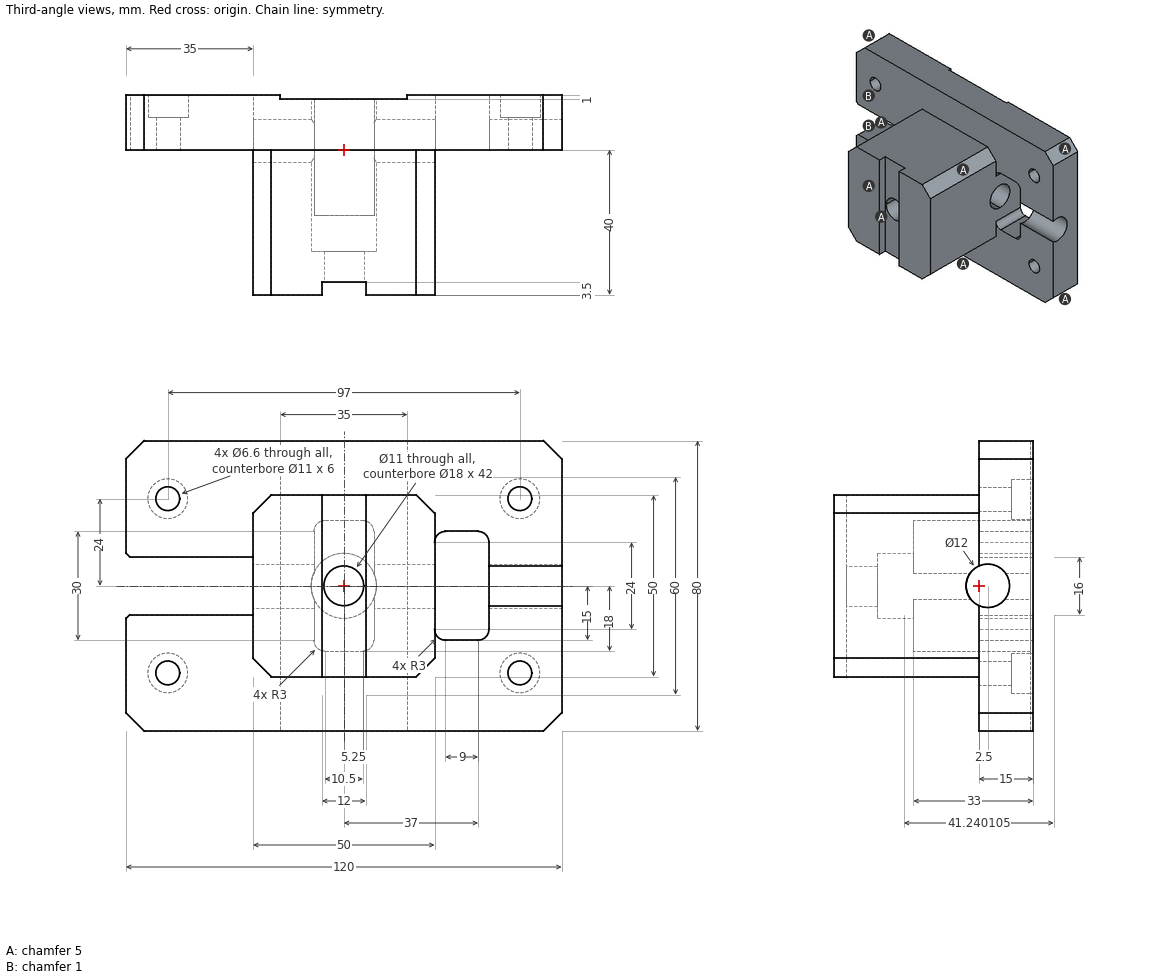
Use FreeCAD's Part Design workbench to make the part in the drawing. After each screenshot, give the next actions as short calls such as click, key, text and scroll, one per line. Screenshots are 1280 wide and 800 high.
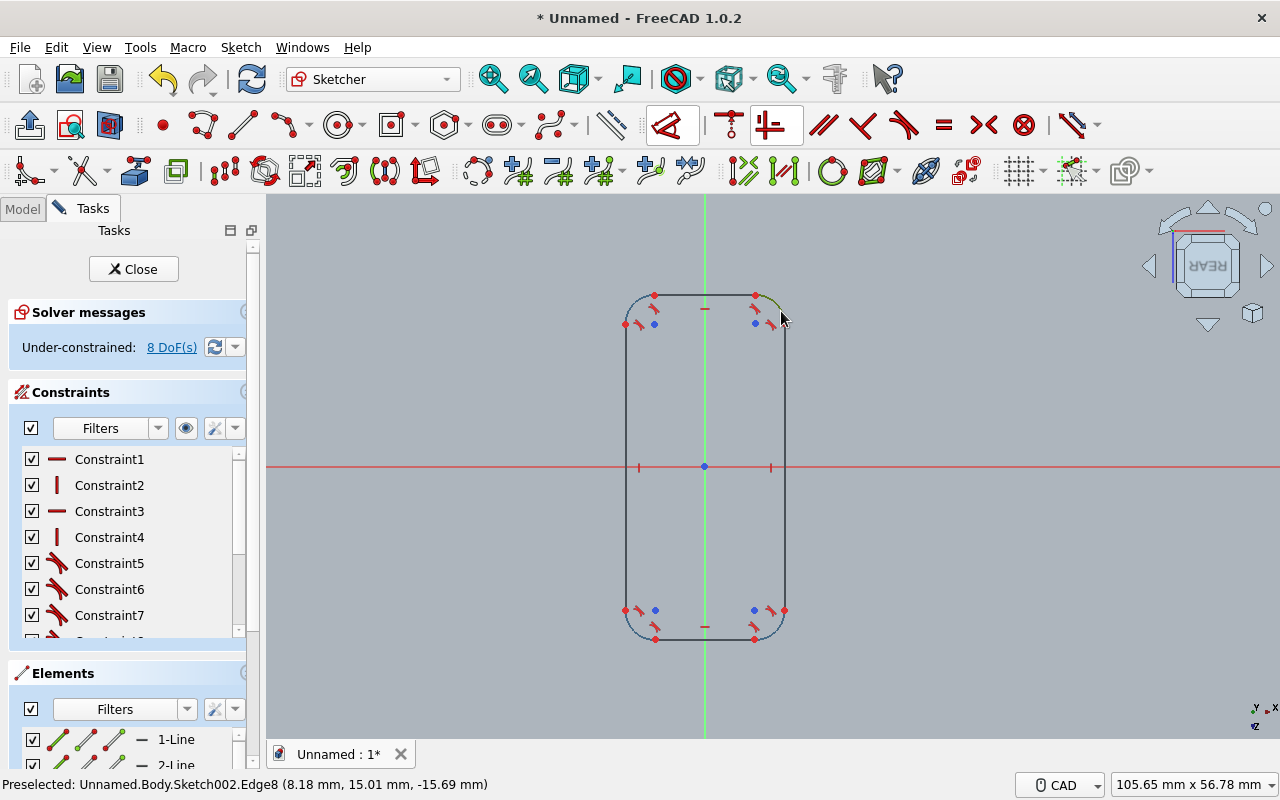
click(944, 126)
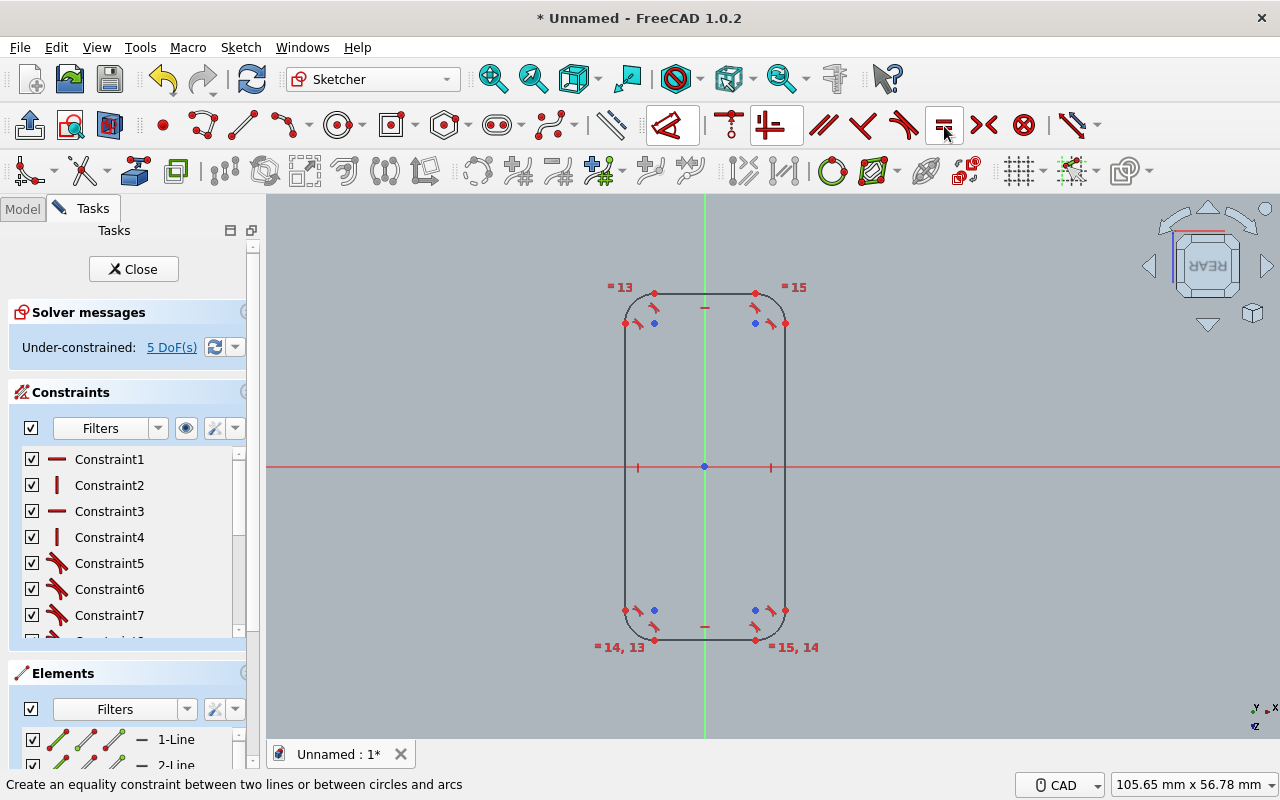
scroll(641, 297, up, 2)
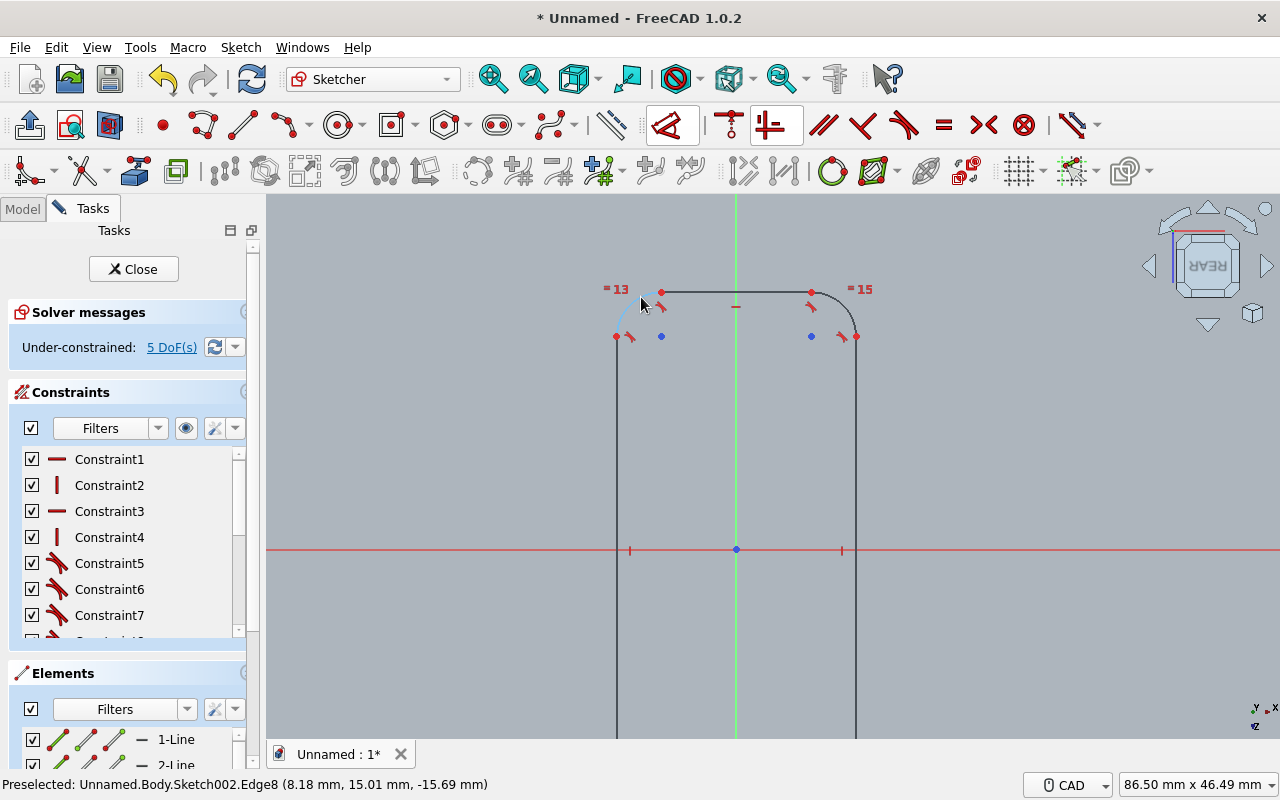
click(641, 297)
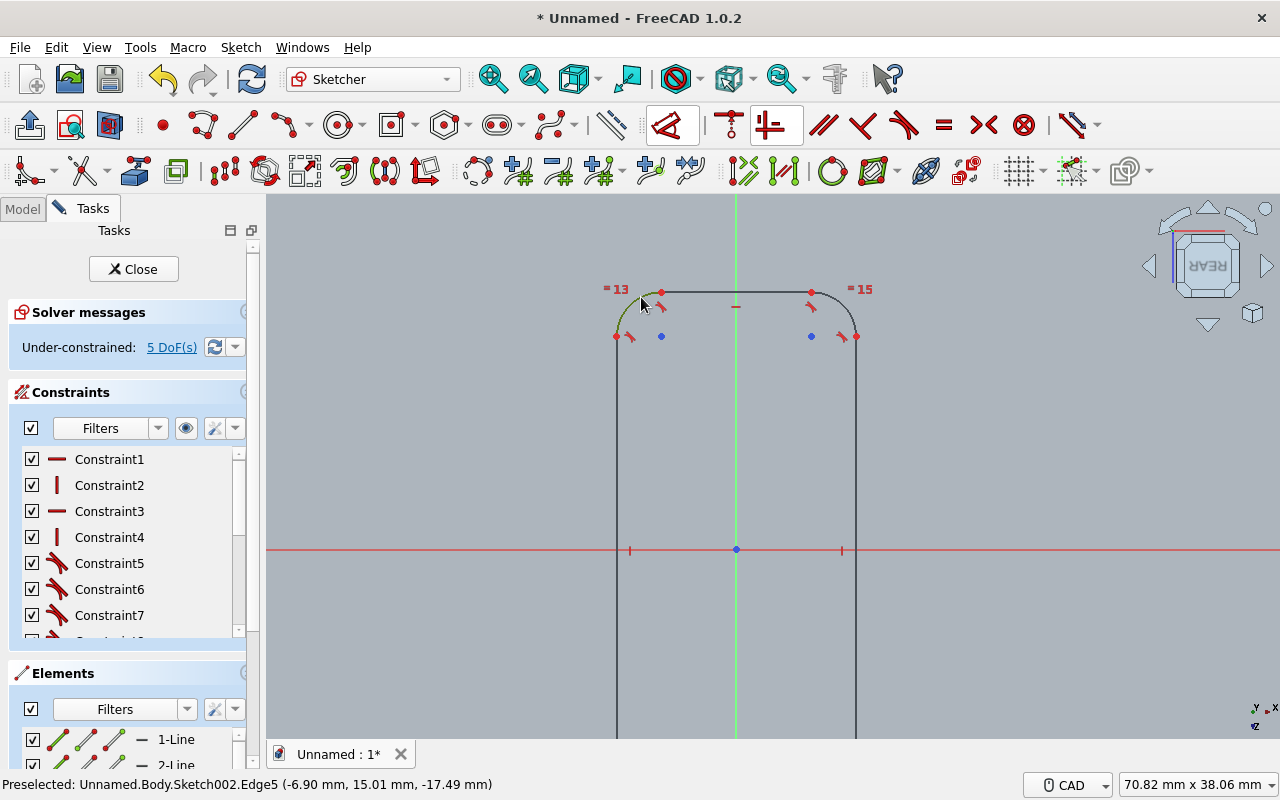
key(k)
key(r)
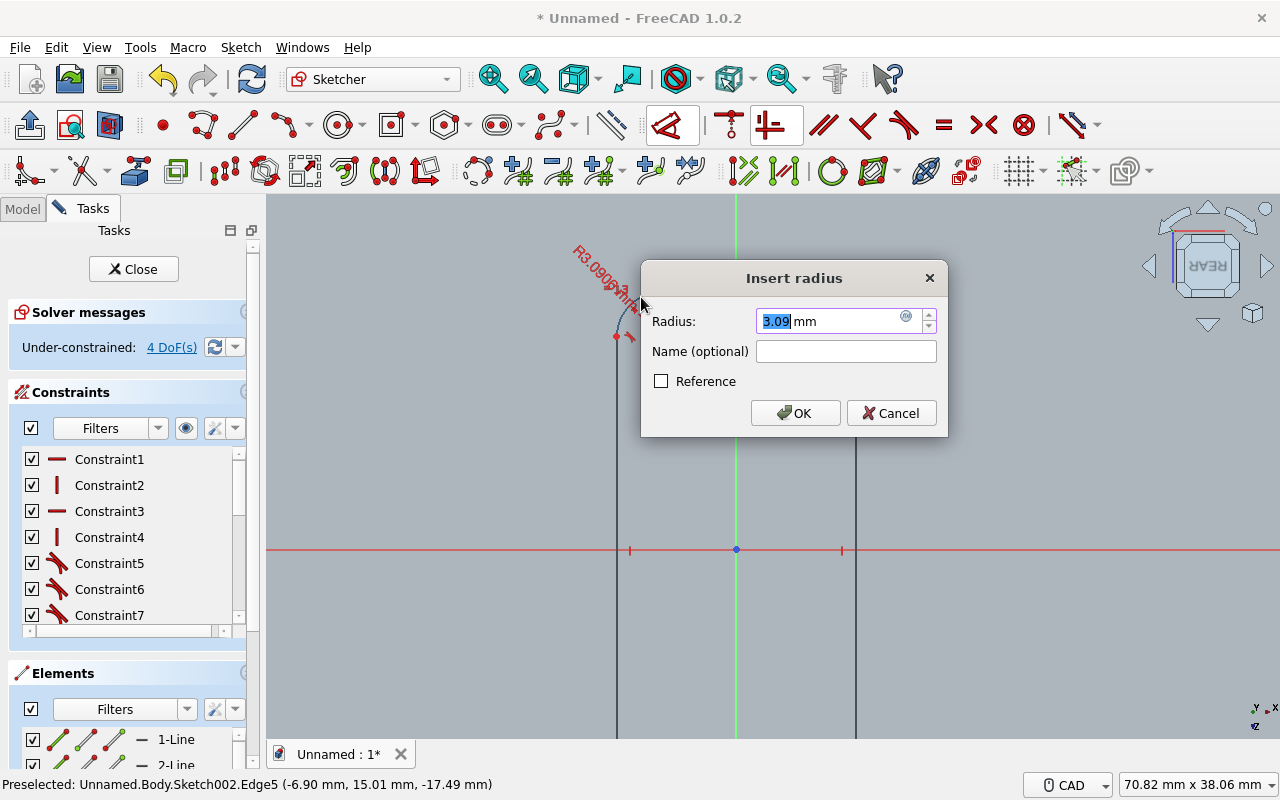
text(3)
key(Return)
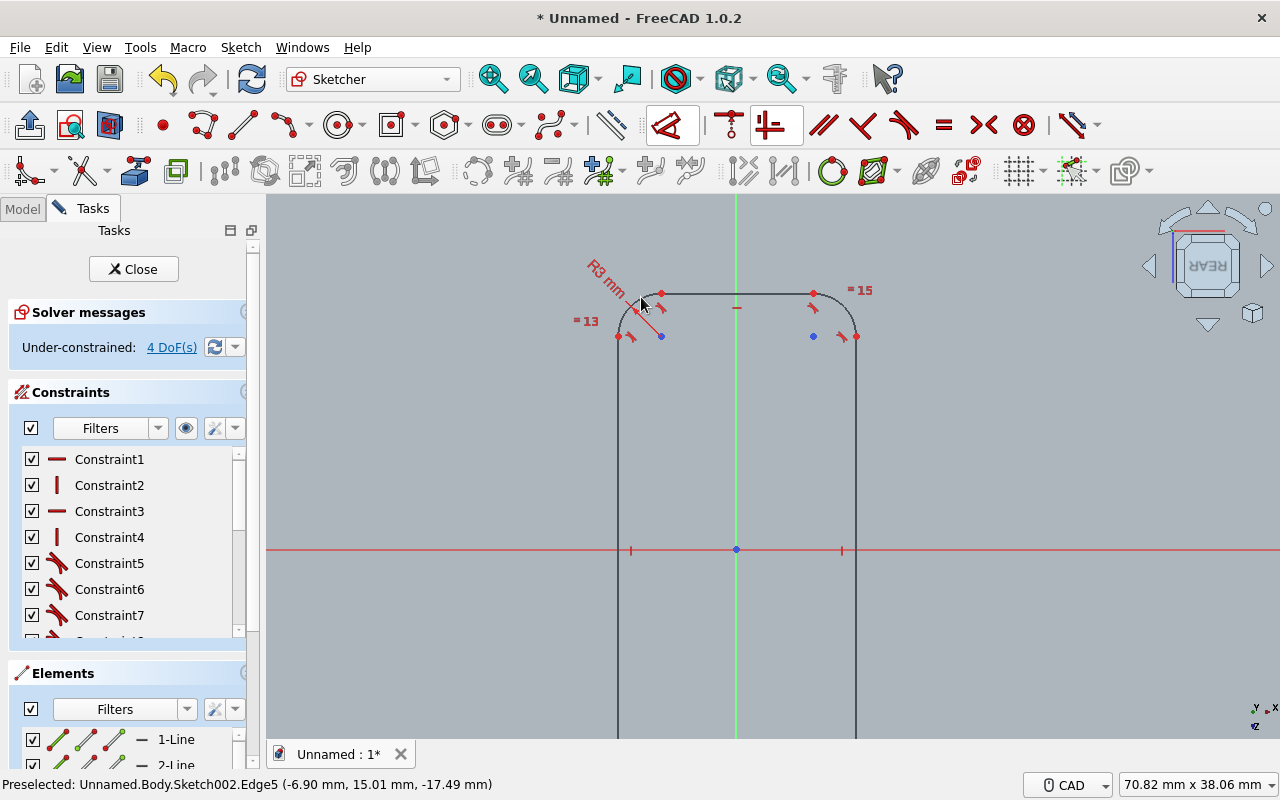
click(618, 465)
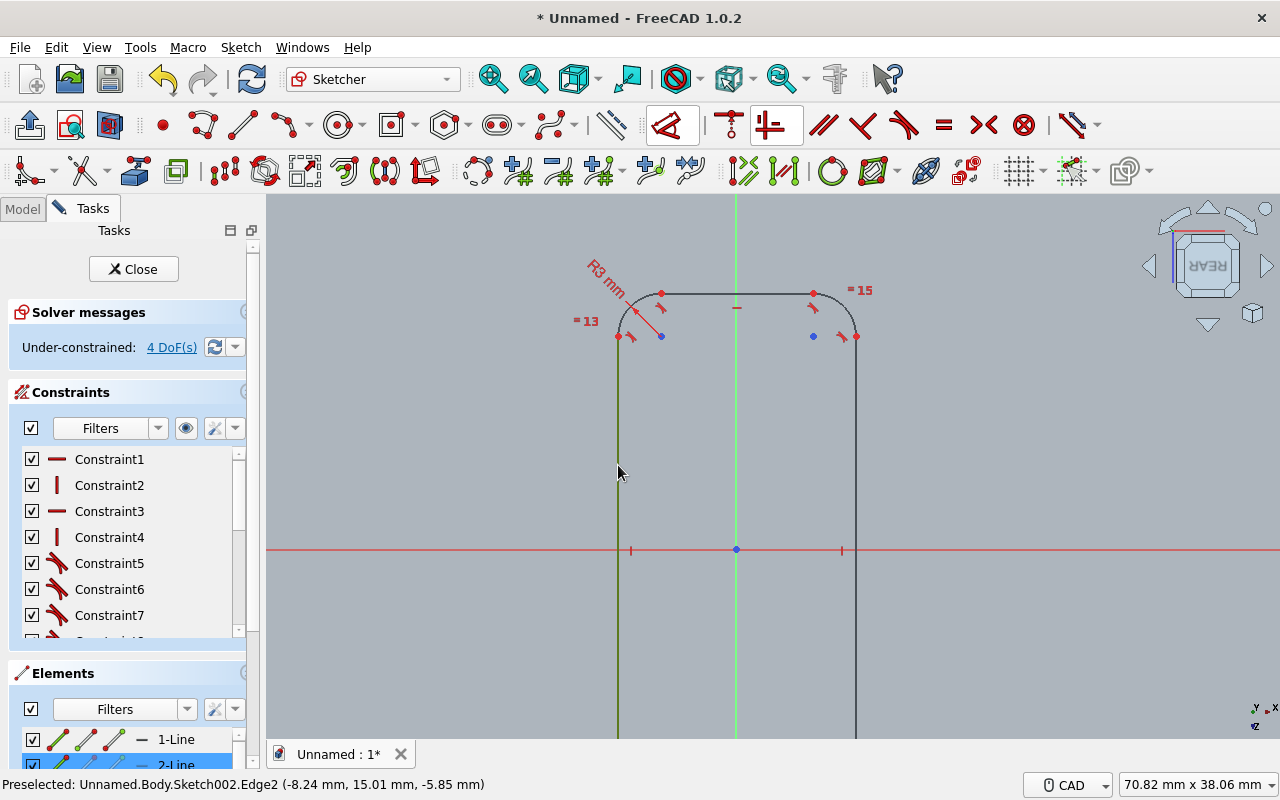
key(i)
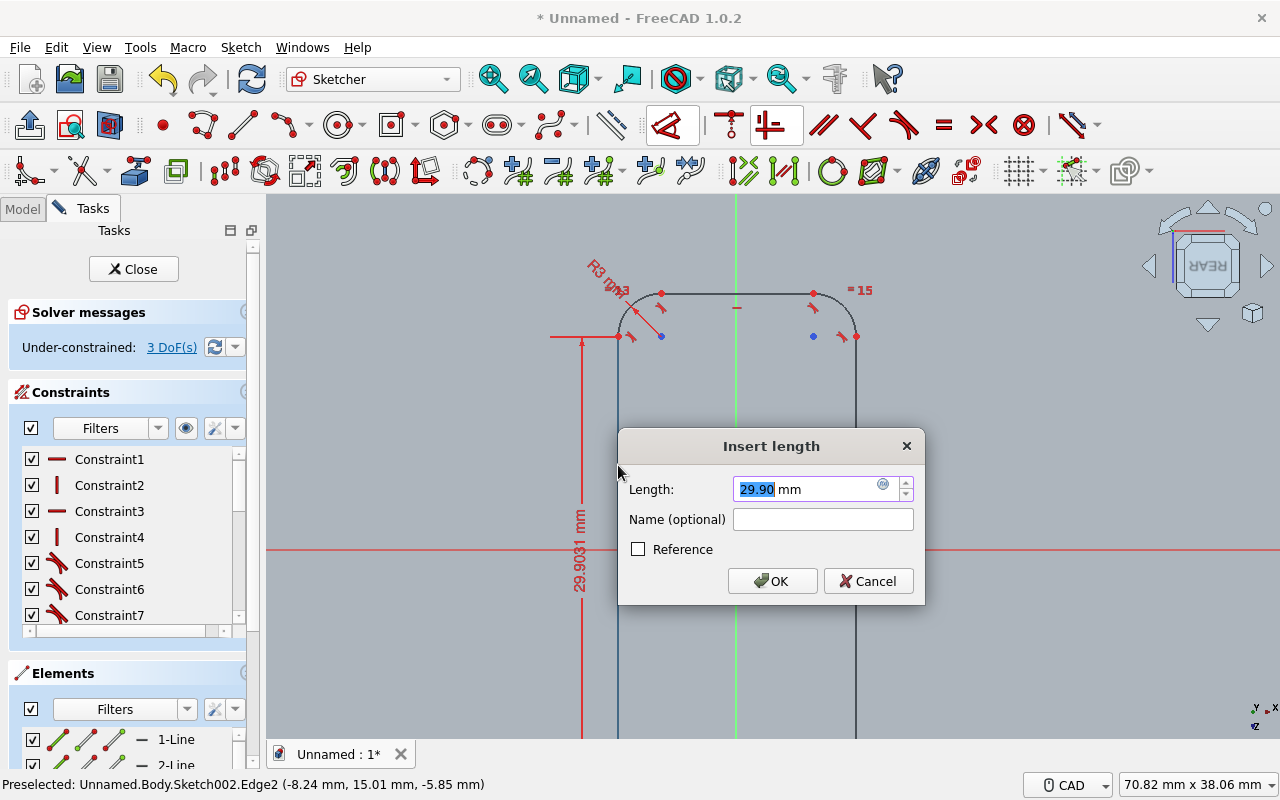
text(30)
key(Return)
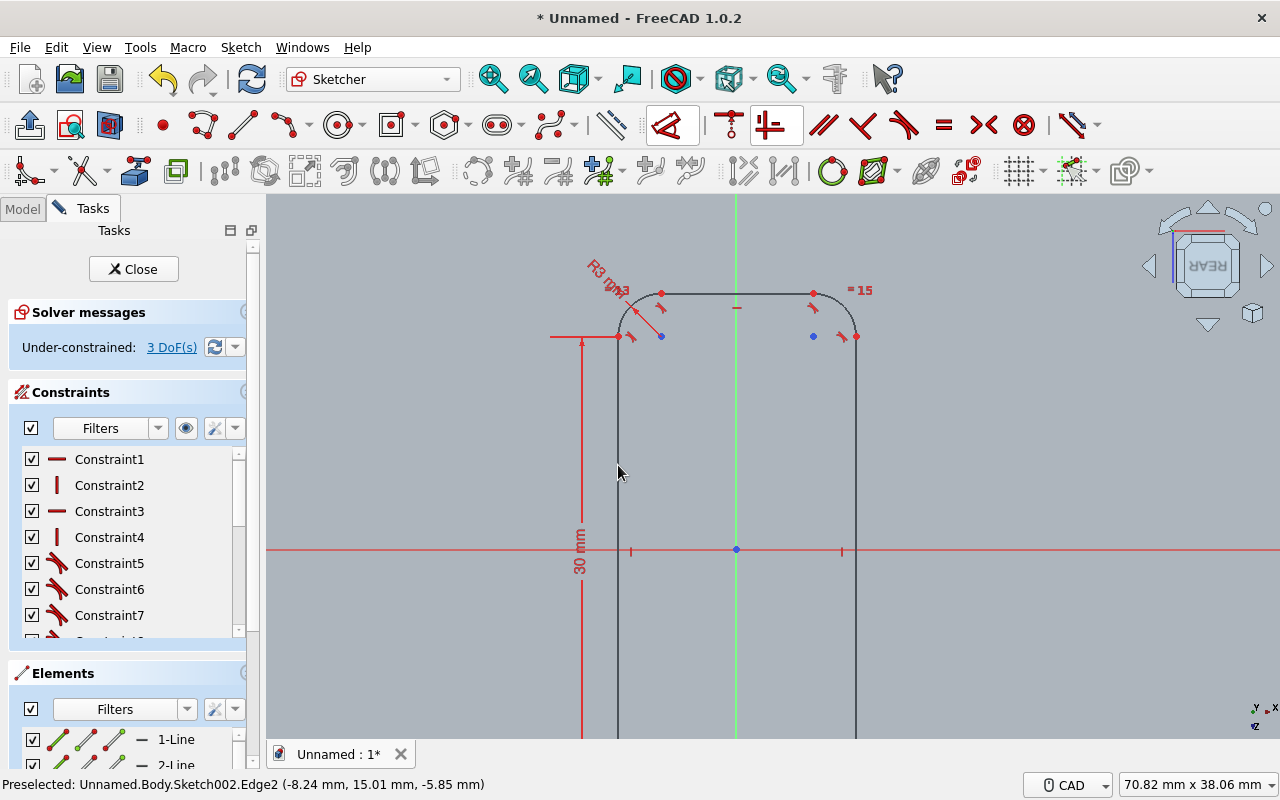
click(813, 294)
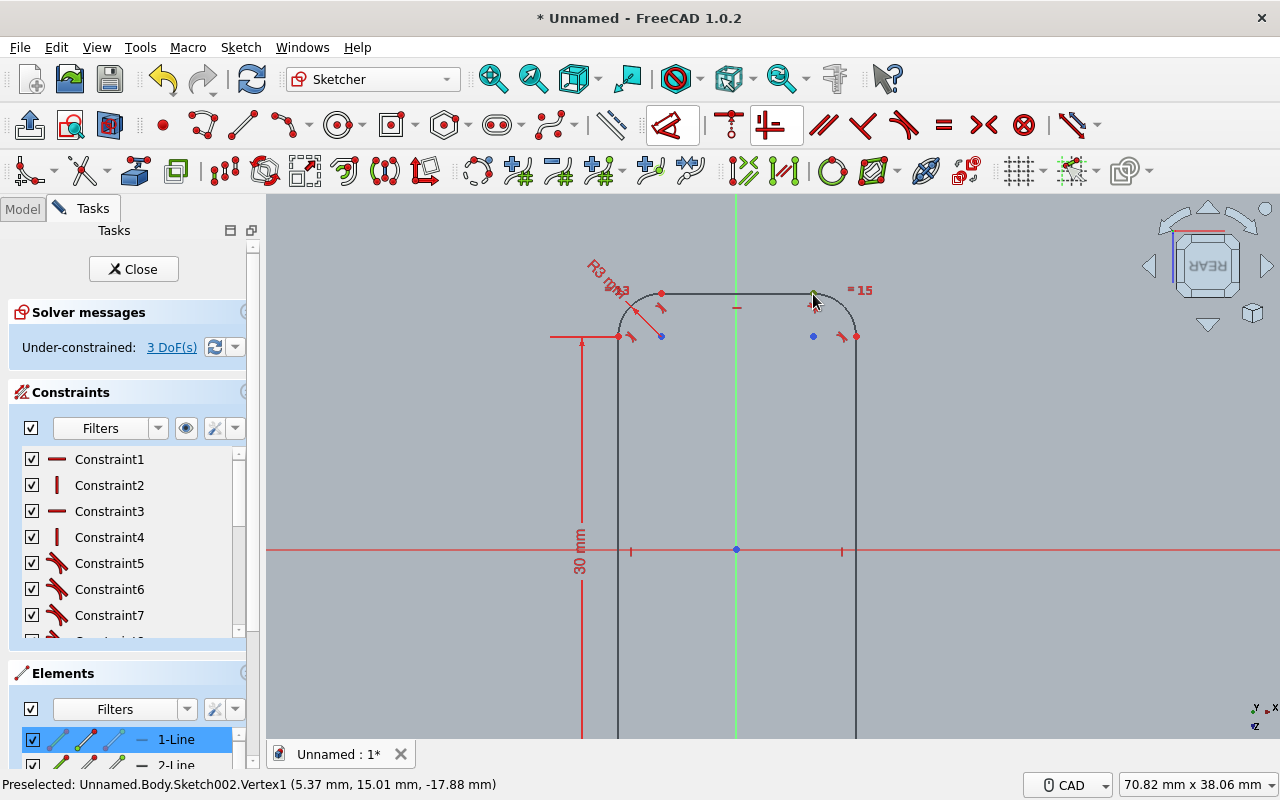
key(i)